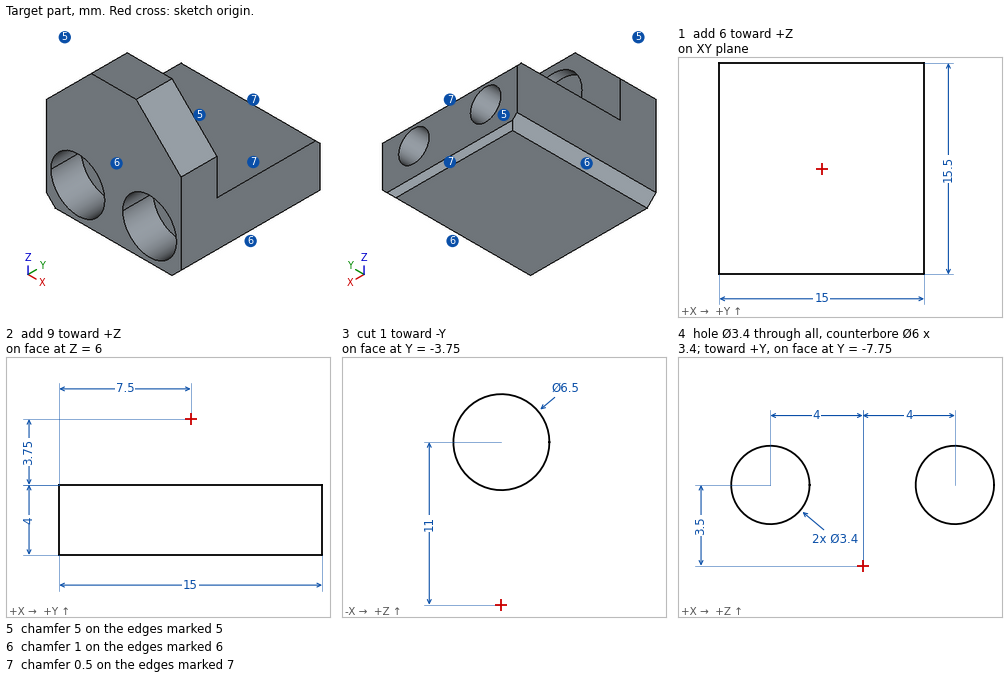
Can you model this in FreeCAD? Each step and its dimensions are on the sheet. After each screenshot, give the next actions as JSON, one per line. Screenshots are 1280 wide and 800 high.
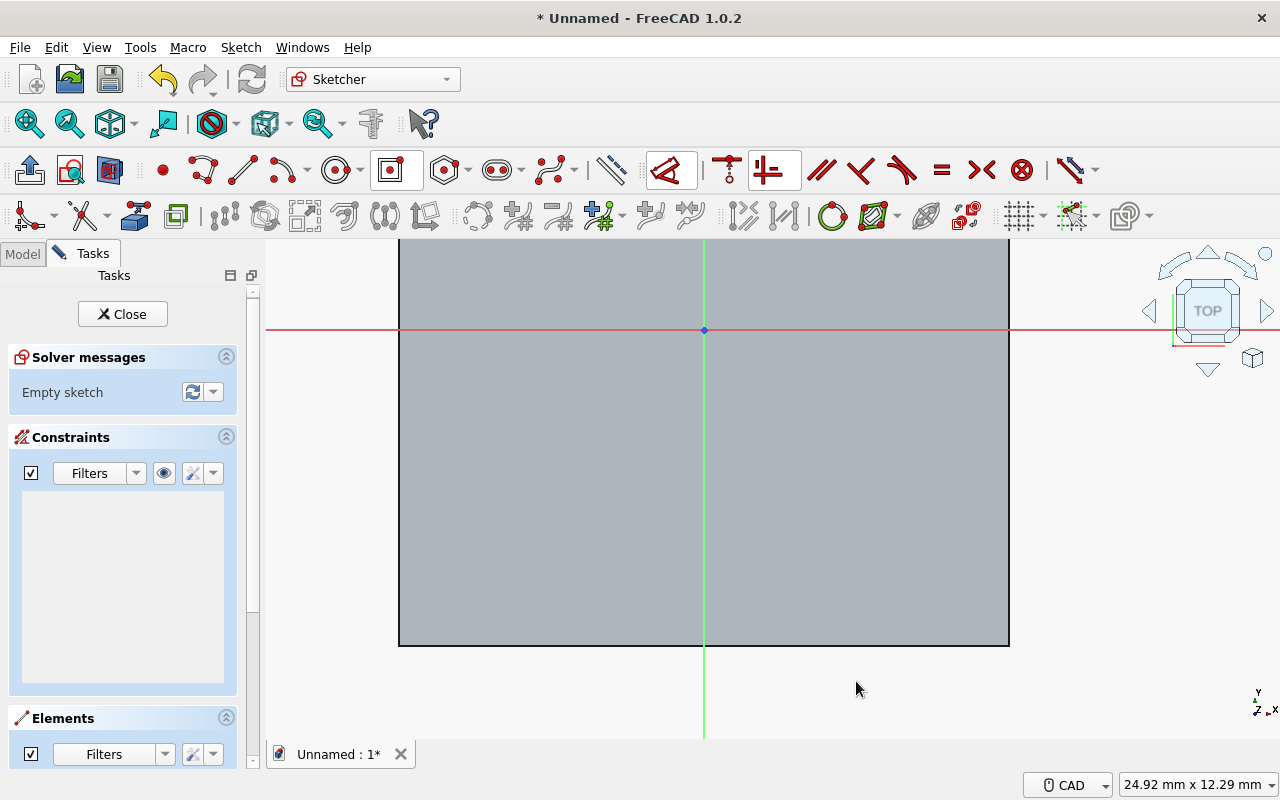
{"action": "key", "text": "g r"}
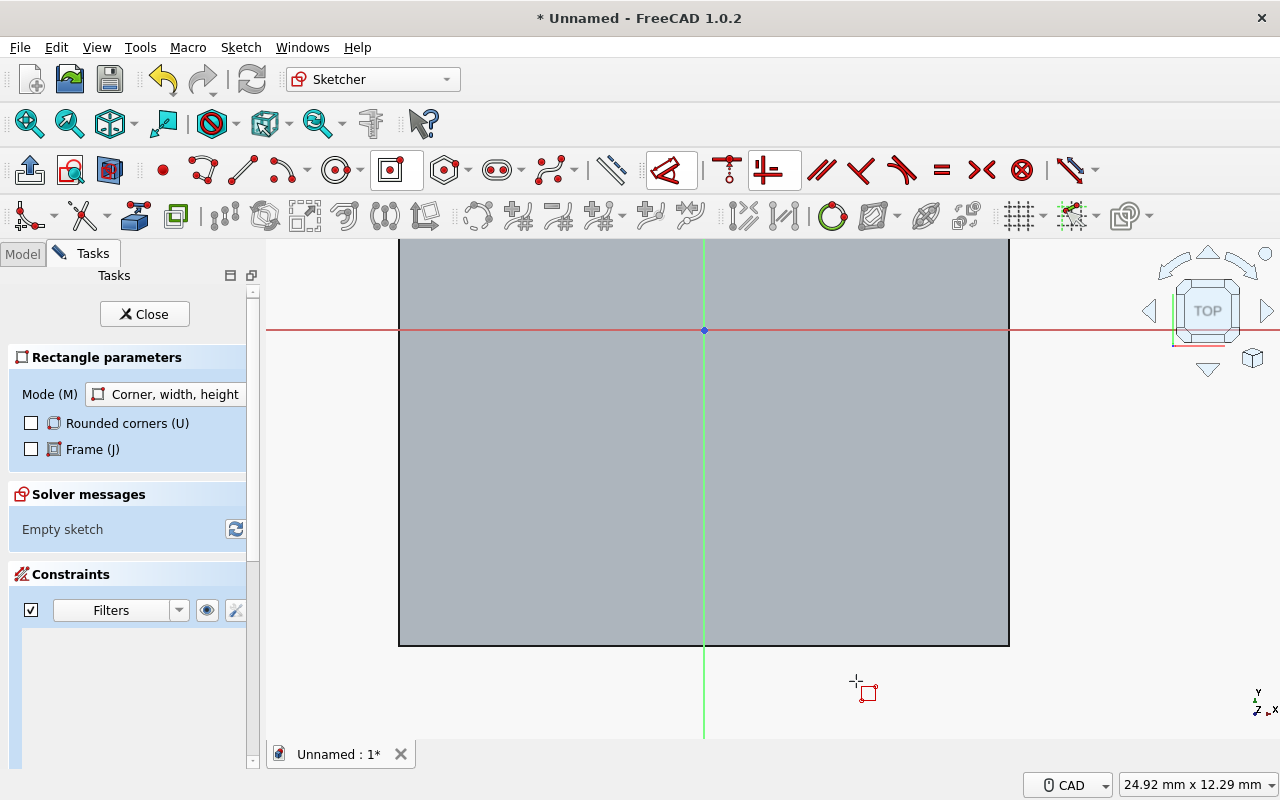
{"action": "left_click", "coordinate": [399, 483]}
{"action": "left_click", "coordinate": [1009, 646]}
{"action": "key", "text": "Escape"}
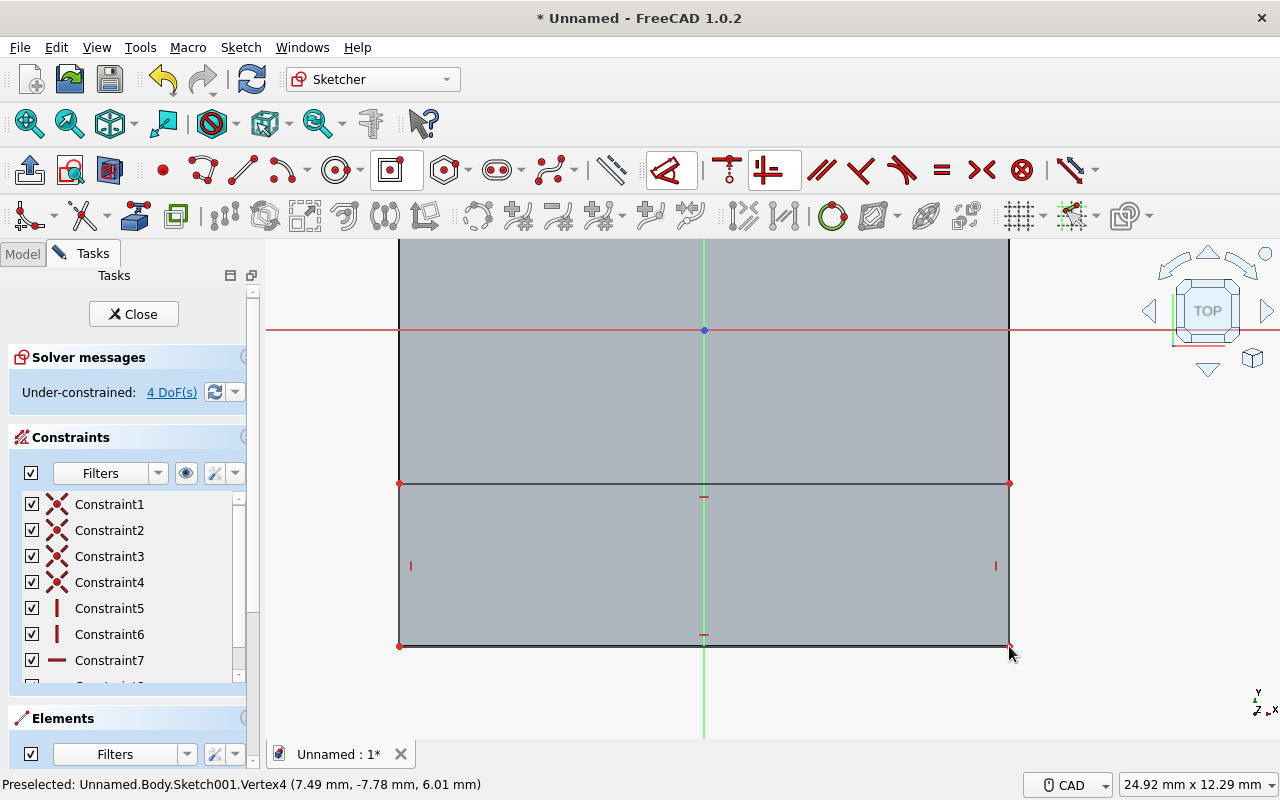
{"action": "key", "text": "d"}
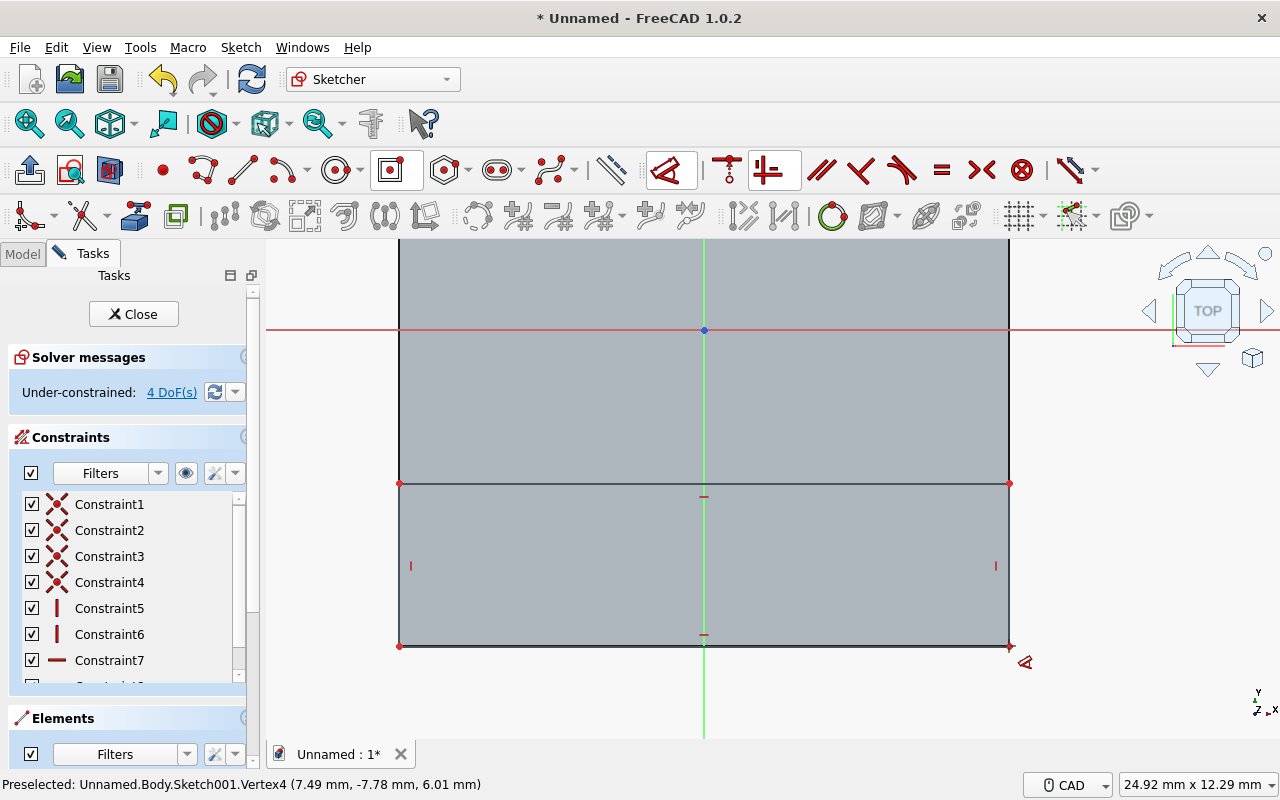
{"action": "left_click", "coordinate": [399, 533]}
{"action": "left_click", "coordinate": [365, 566]}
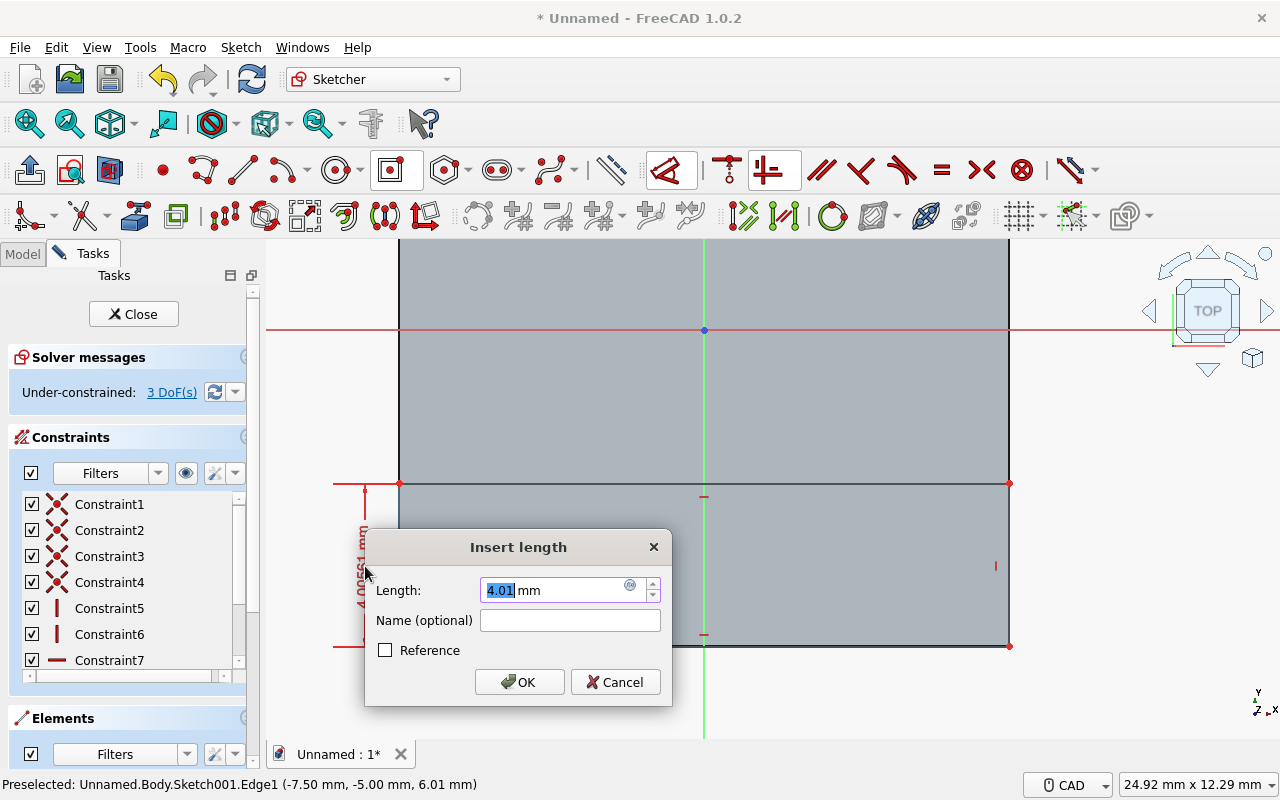
{"action": "type", "text": "4"}
{"action": "key", "text": "Return"}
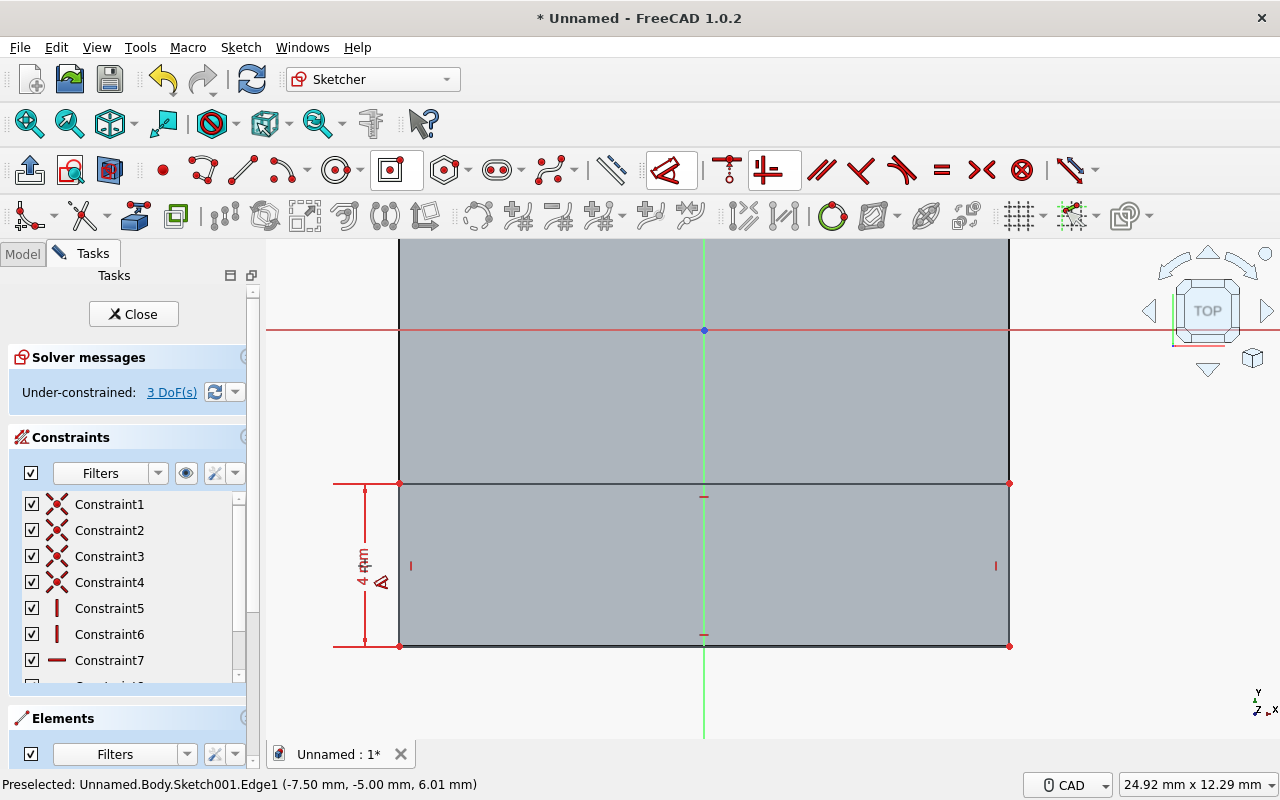
{"action": "left_click", "coordinate": [582, 647]}
{"action": "left_click", "coordinate": [564, 681]}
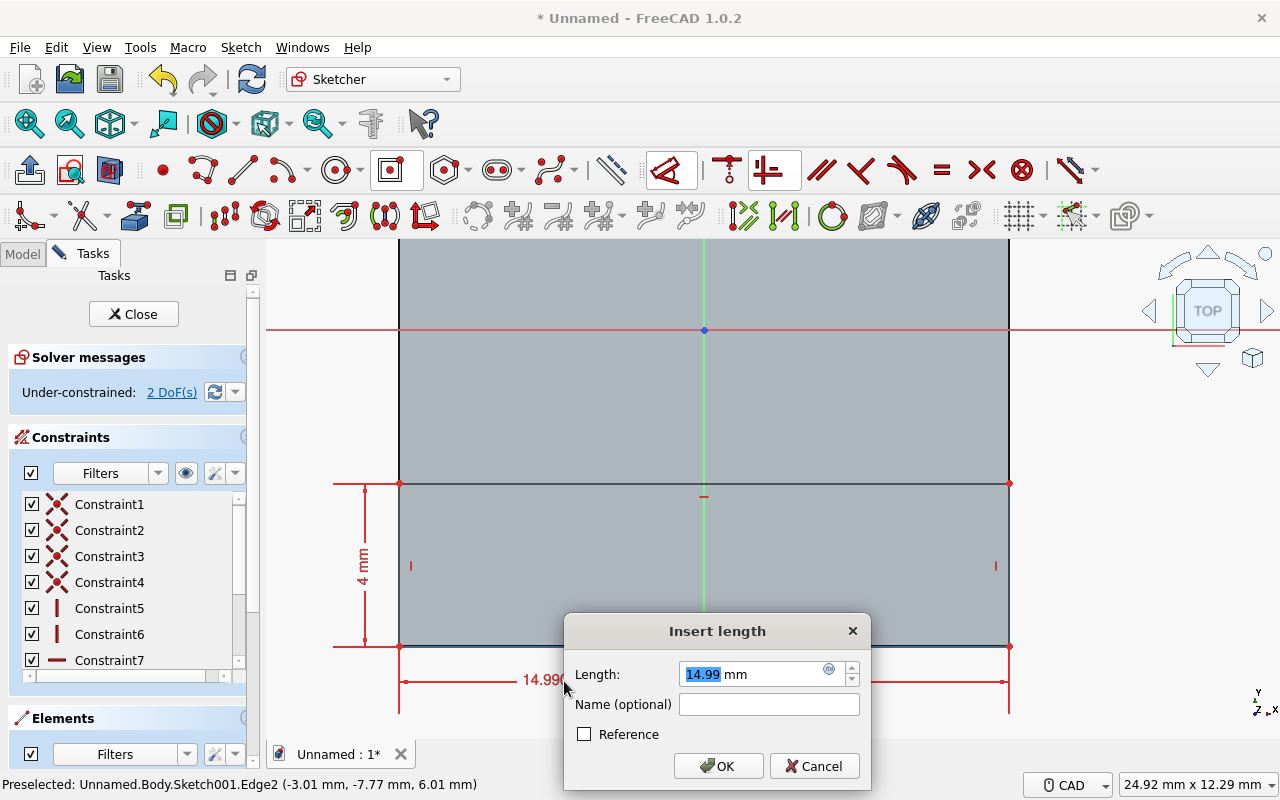
{"action": "type", "text": "15"}
{"action": "key", "text": "Return"}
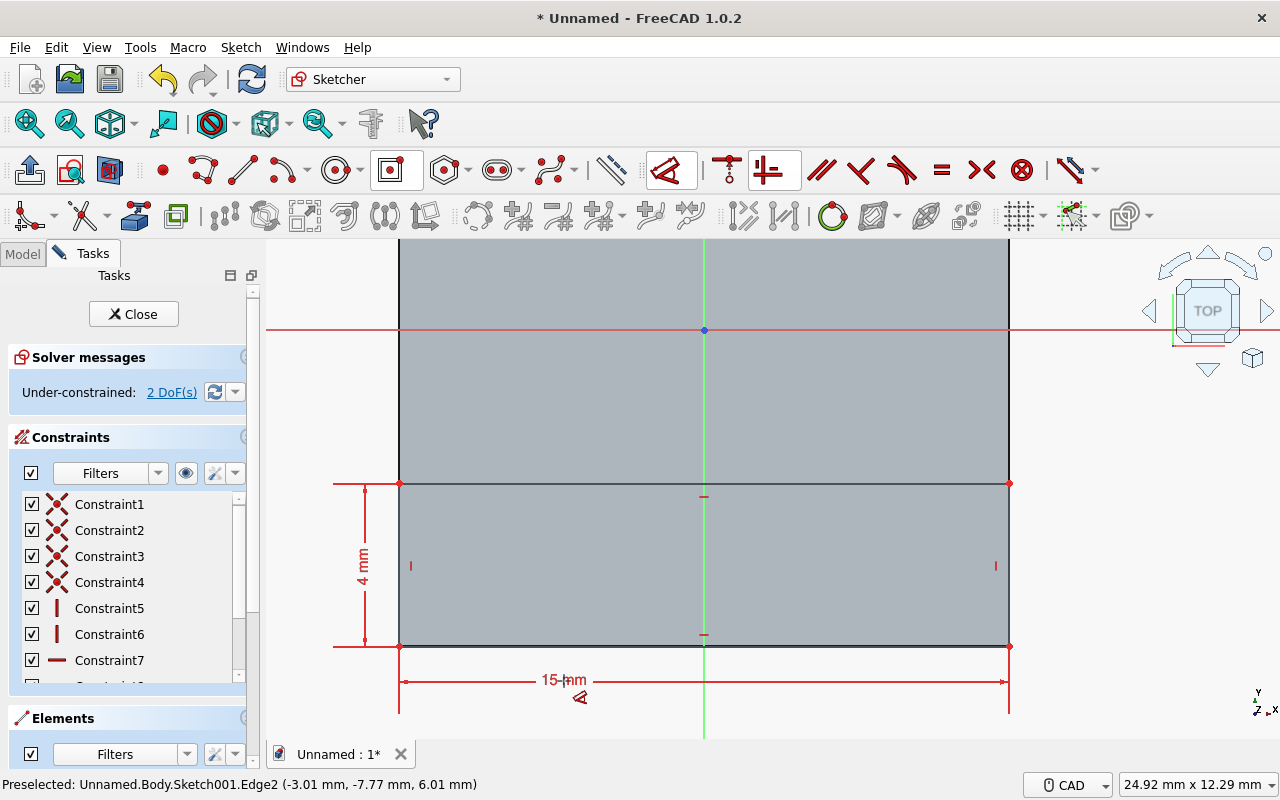
{"action": "left_click", "coordinate": [399, 484]}
{"action": "left_click", "coordinate": [552, 296]}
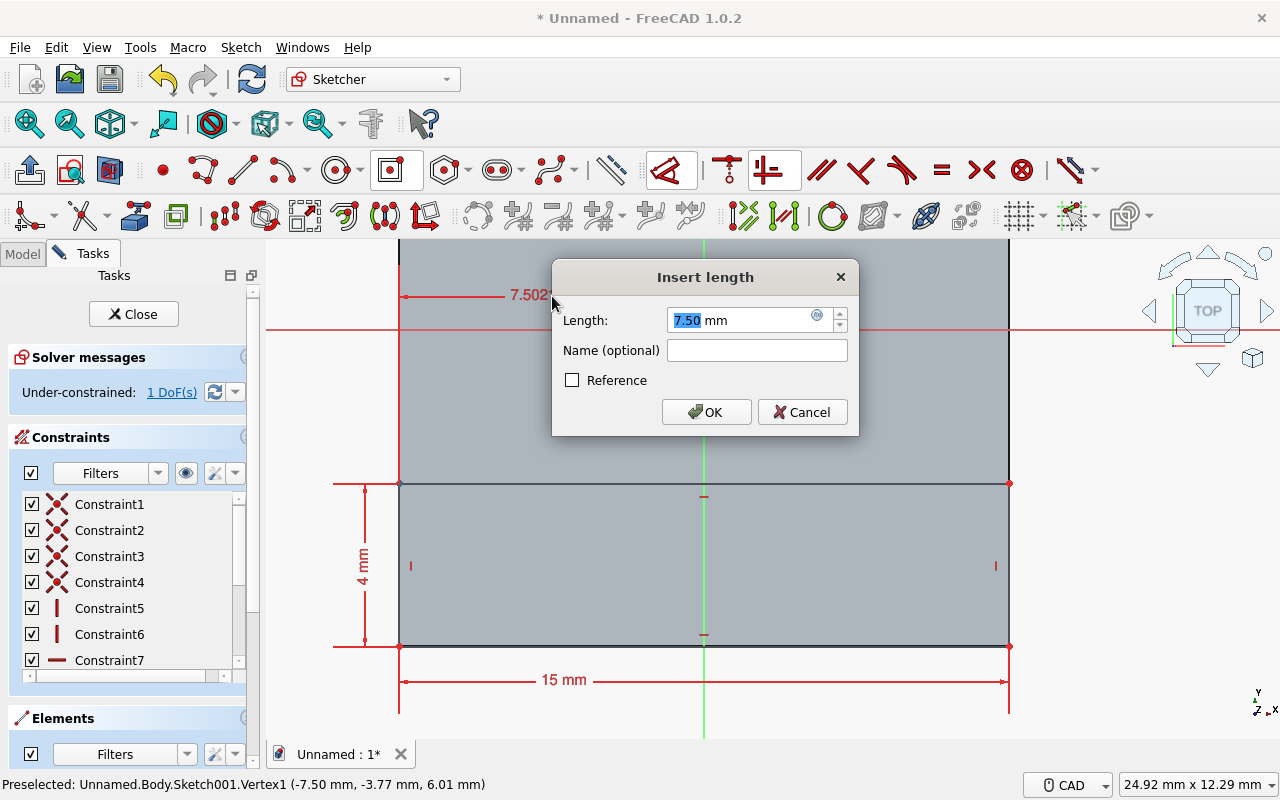
{"action": "type", "text": "7.5"}
{"action": "key", "text": "Return"}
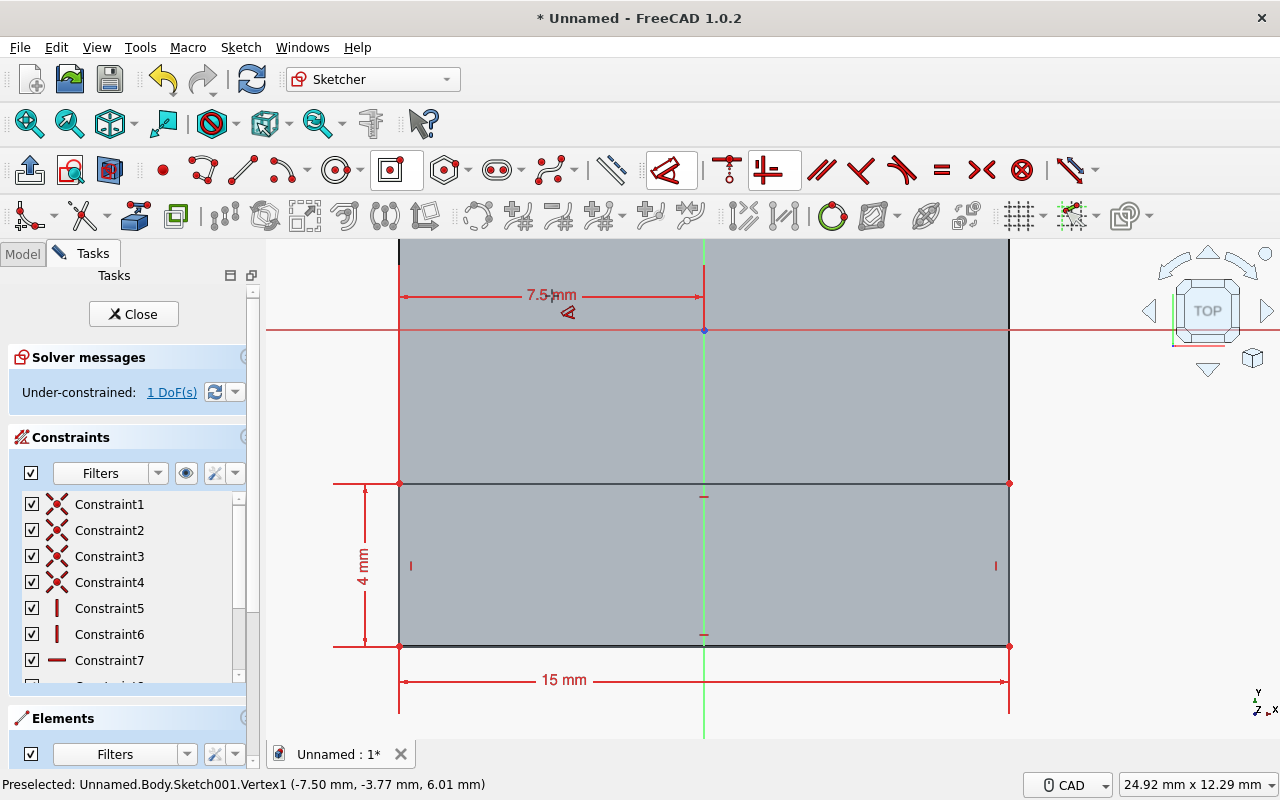
{"action": "left_click", "coordinate": [399, 484]}
{"action": "left_click", "coordinate": [365, 407]}